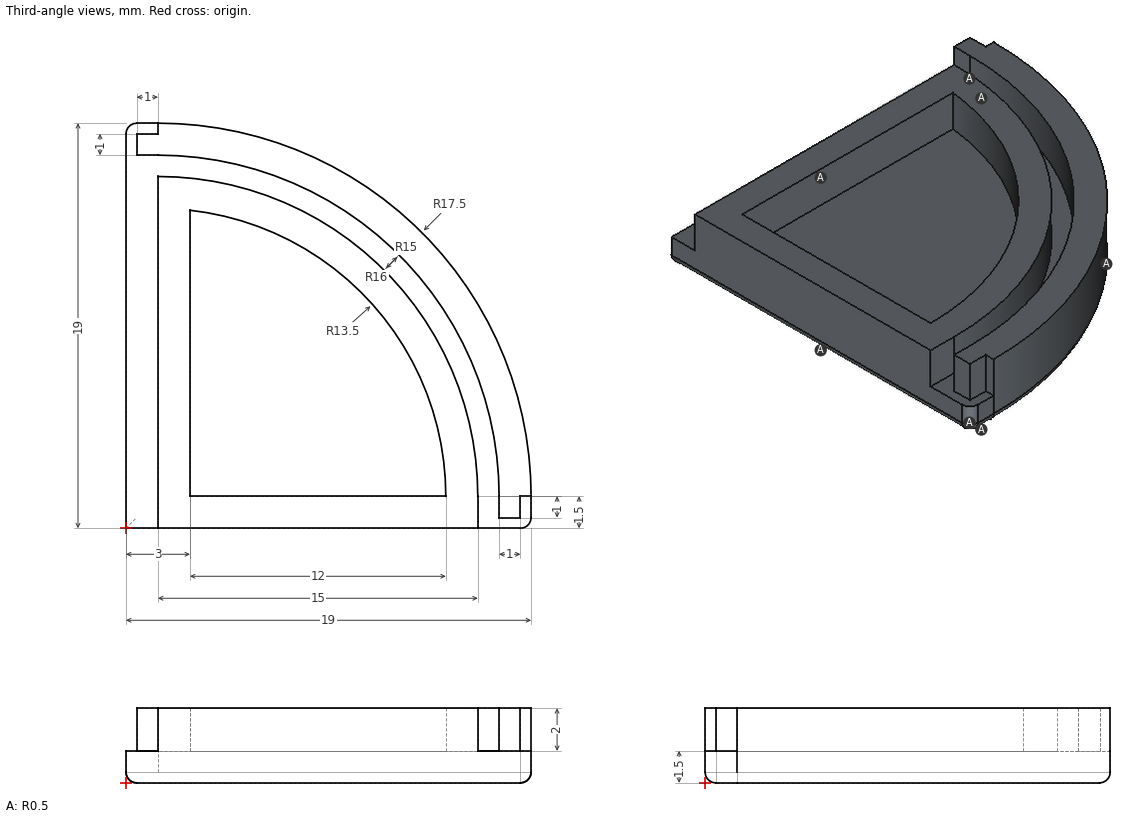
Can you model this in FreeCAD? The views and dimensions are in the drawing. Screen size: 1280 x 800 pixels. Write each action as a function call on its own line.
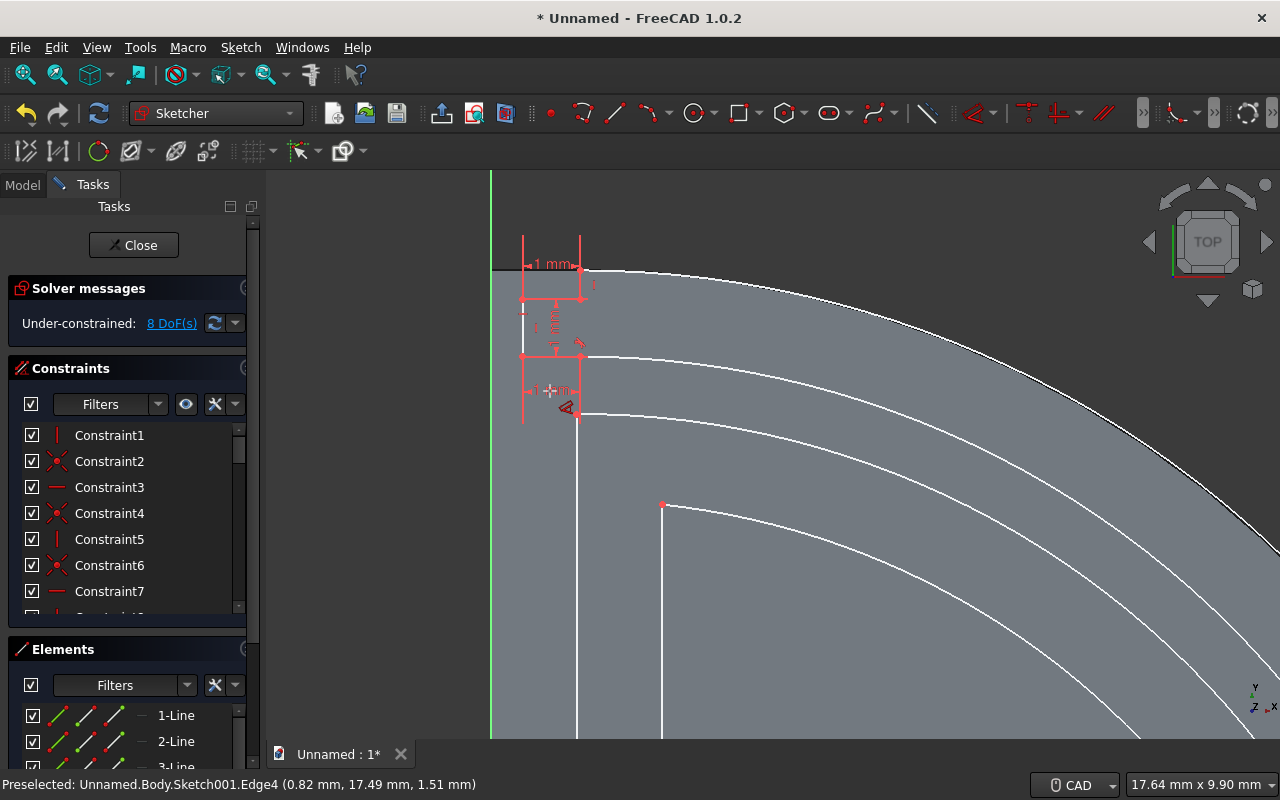
scroll(561, 299, down, 6)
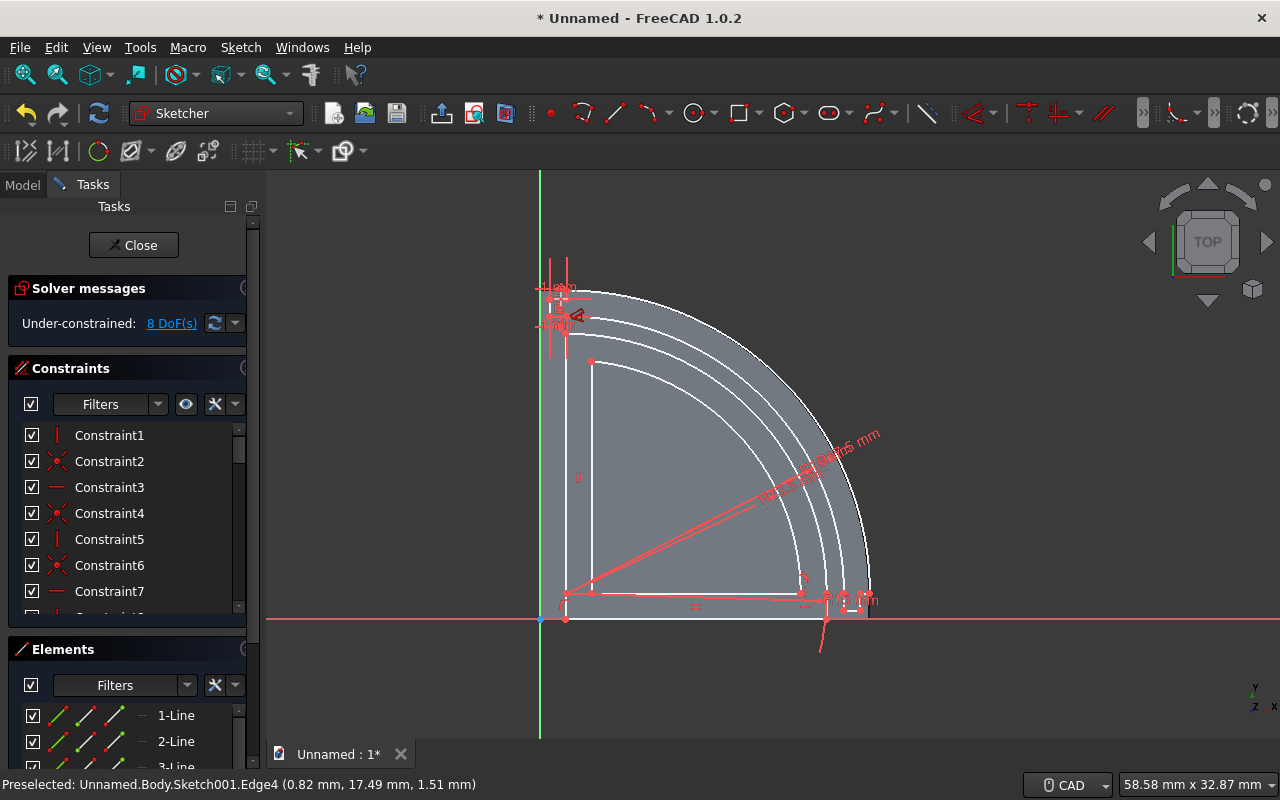
scroll(844, 599, up, 5)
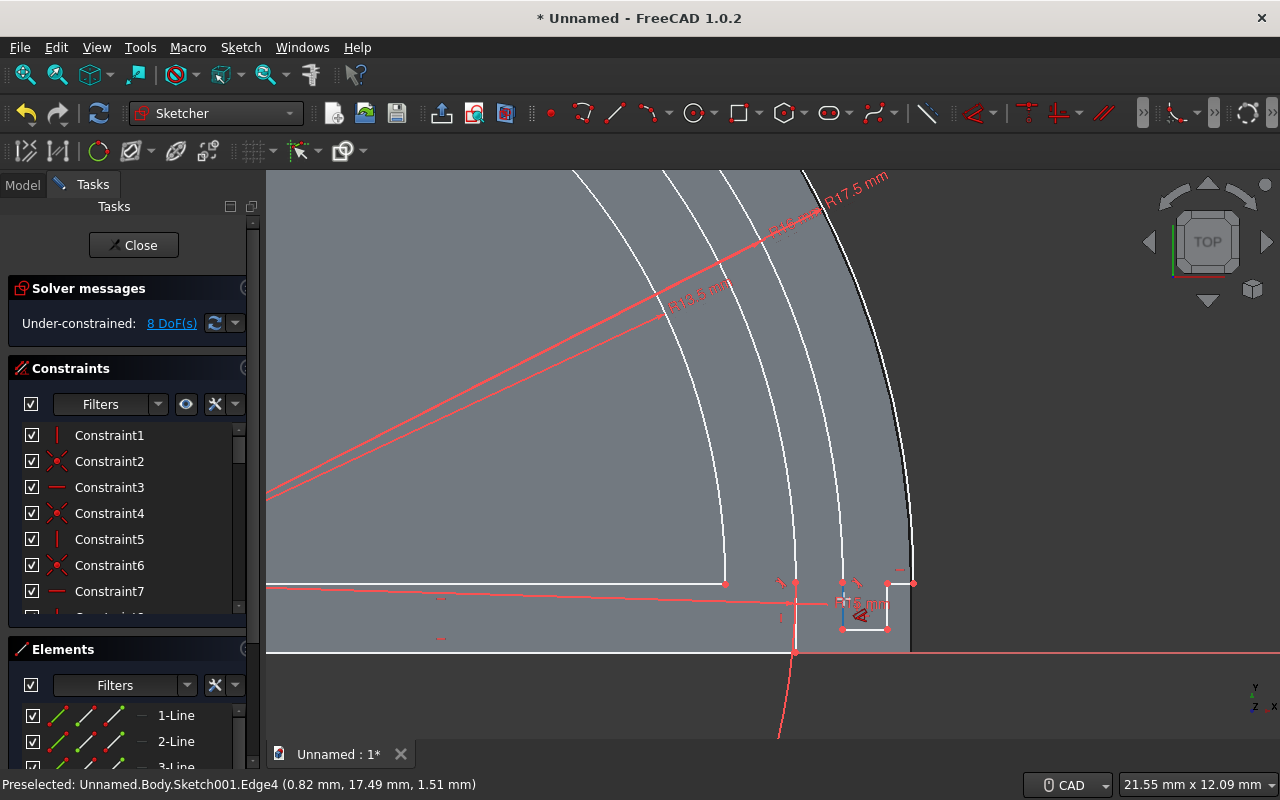
click(843, 597)
click(761, 606)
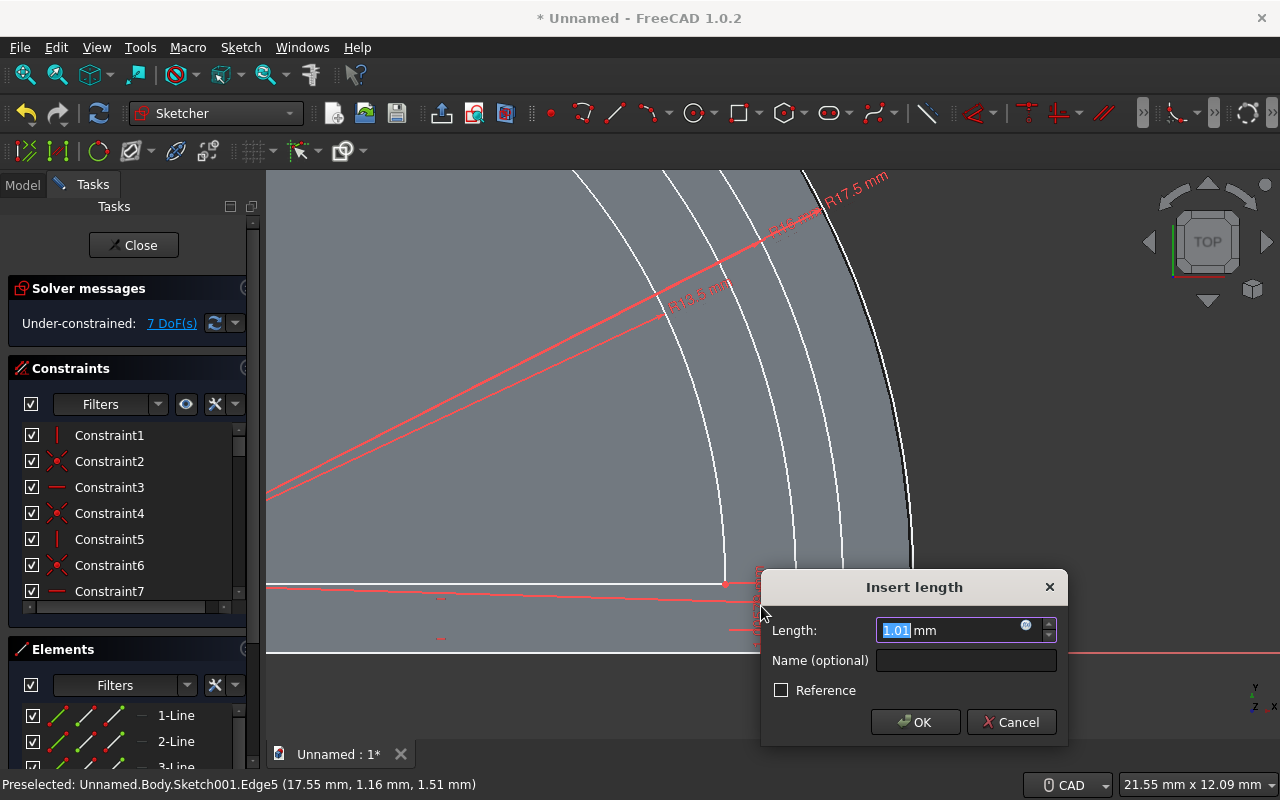
text(1)
key(Return)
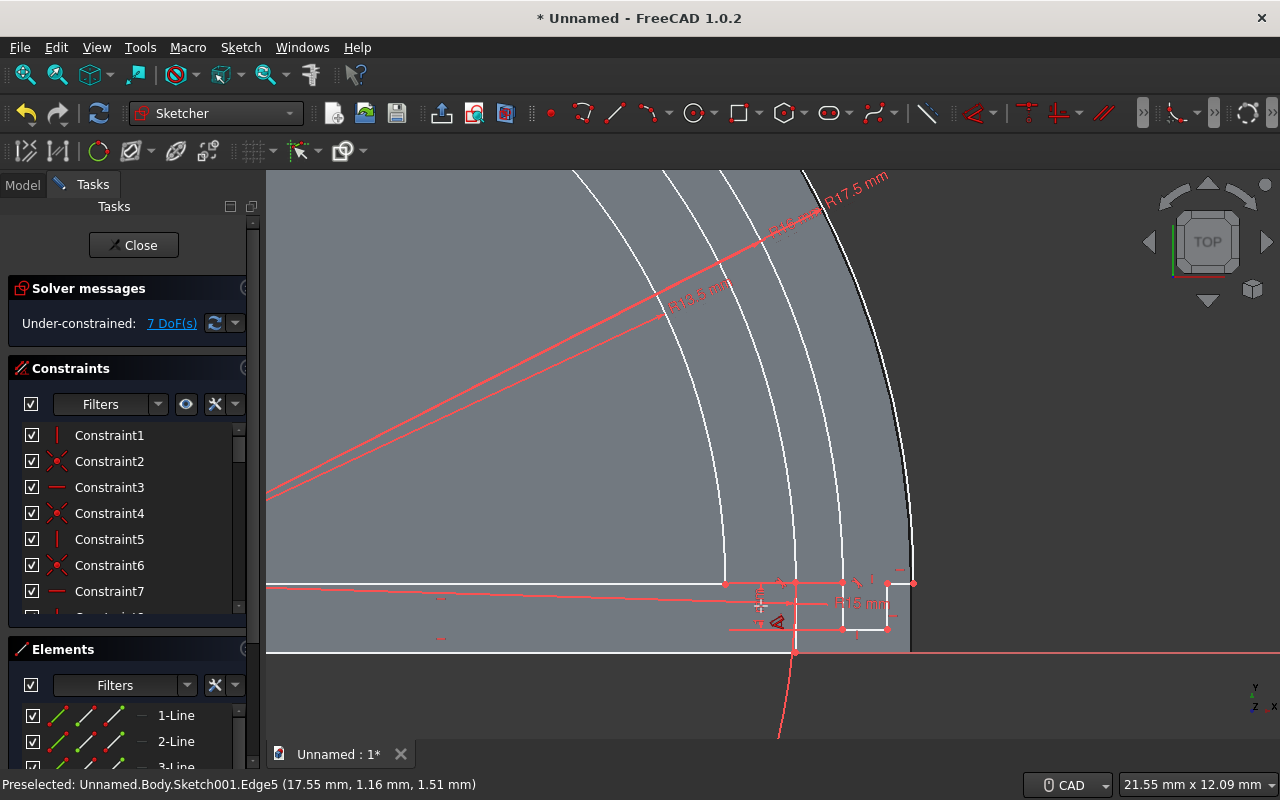
click(856, 630)
click(865, 688)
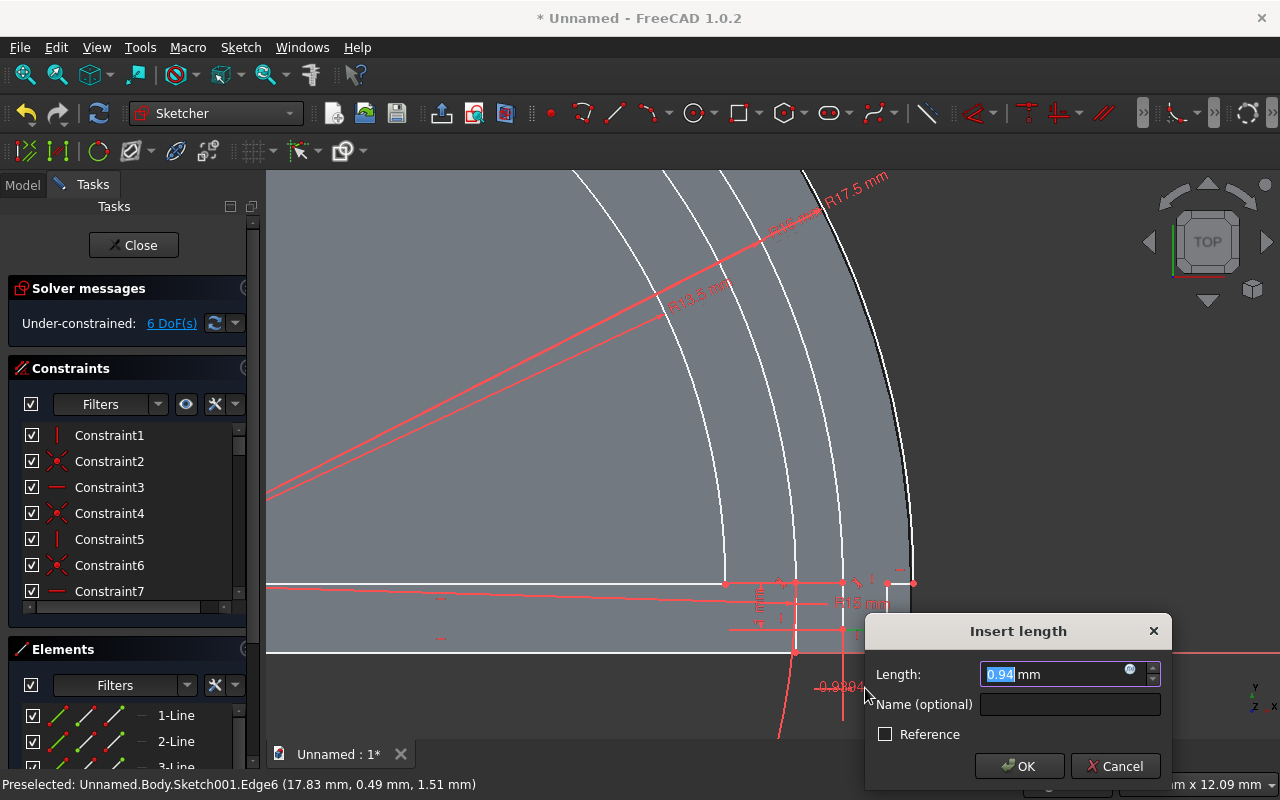
text(1)
key(Return)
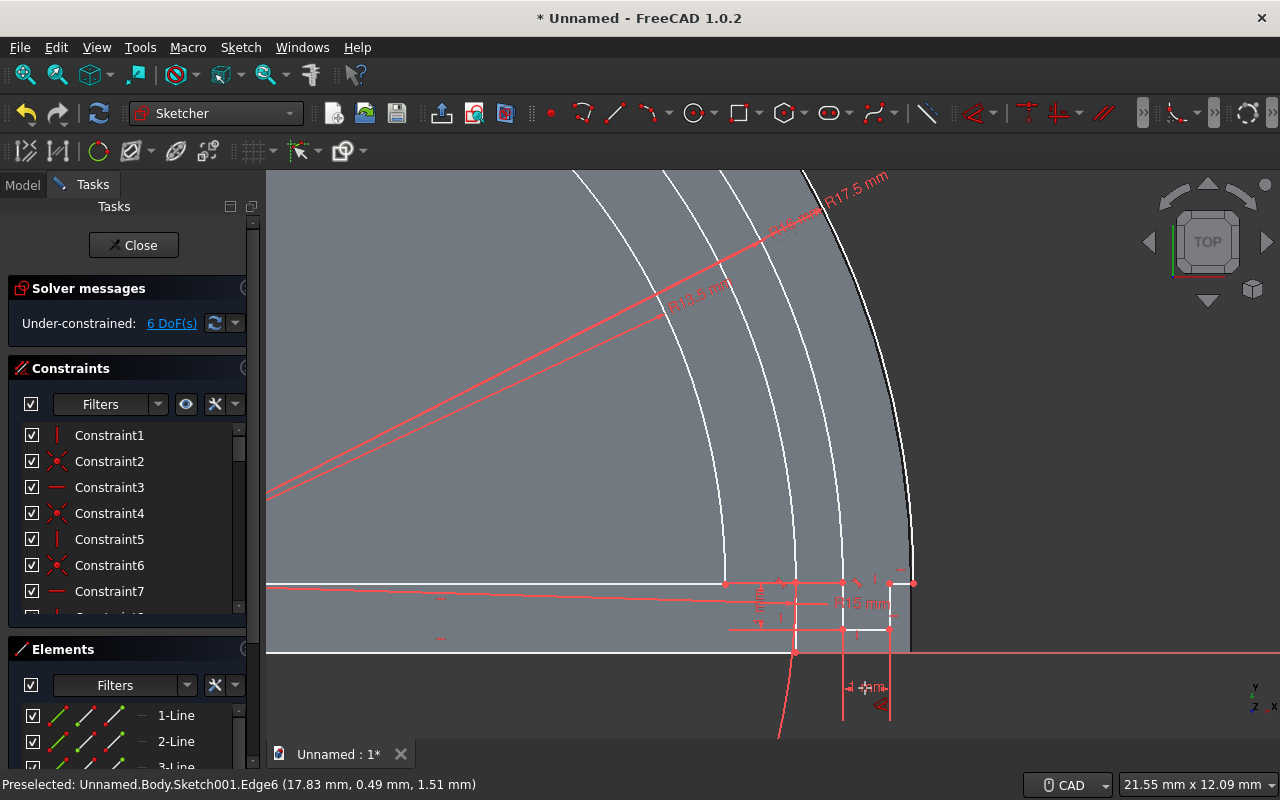
click(890, 616)
click(948, 607)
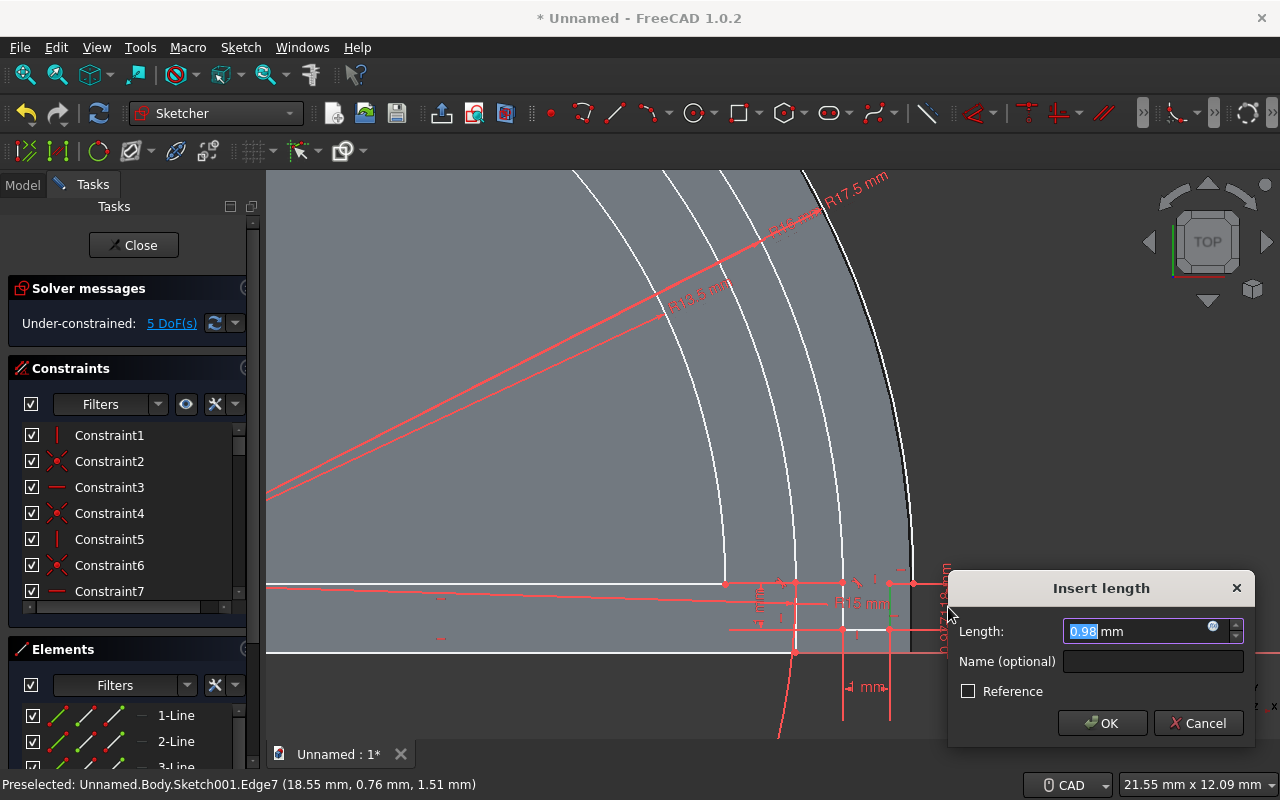
text(1)
key(Return)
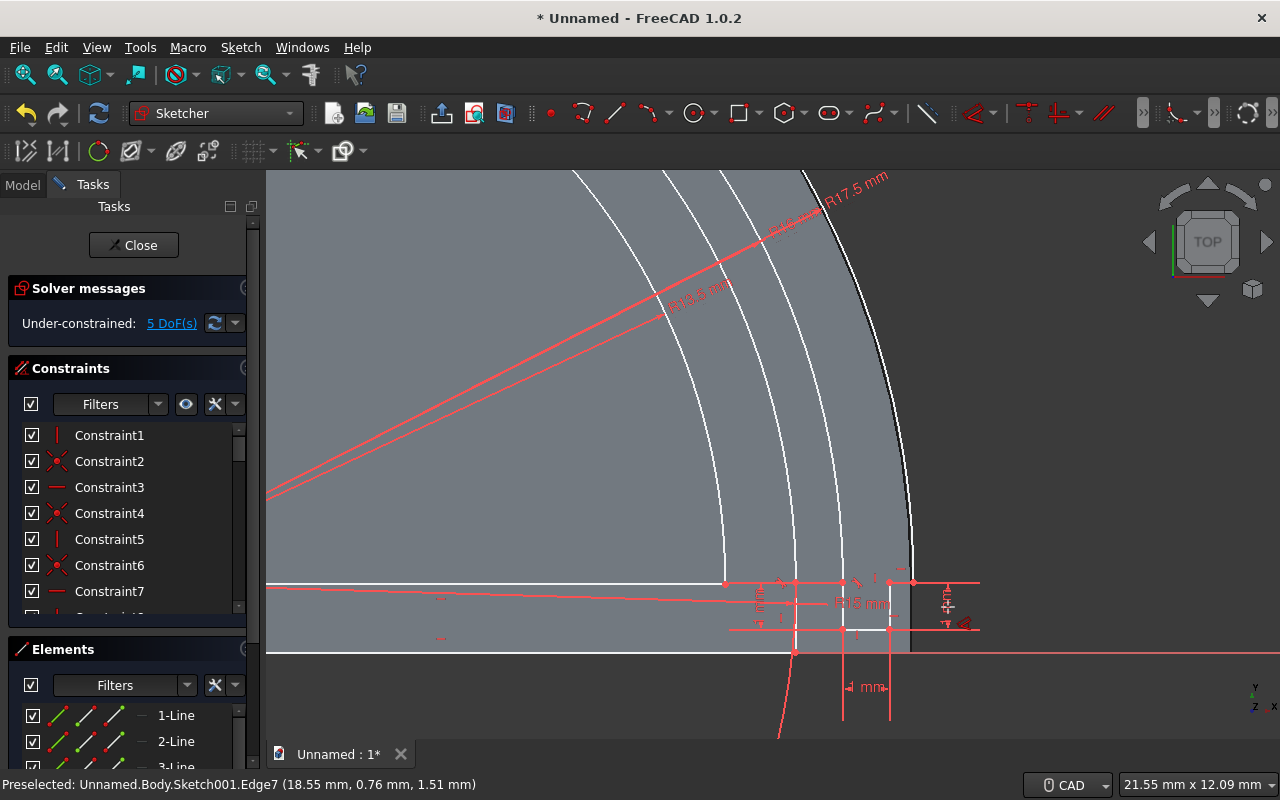
click(300, 653)
click(545, 687)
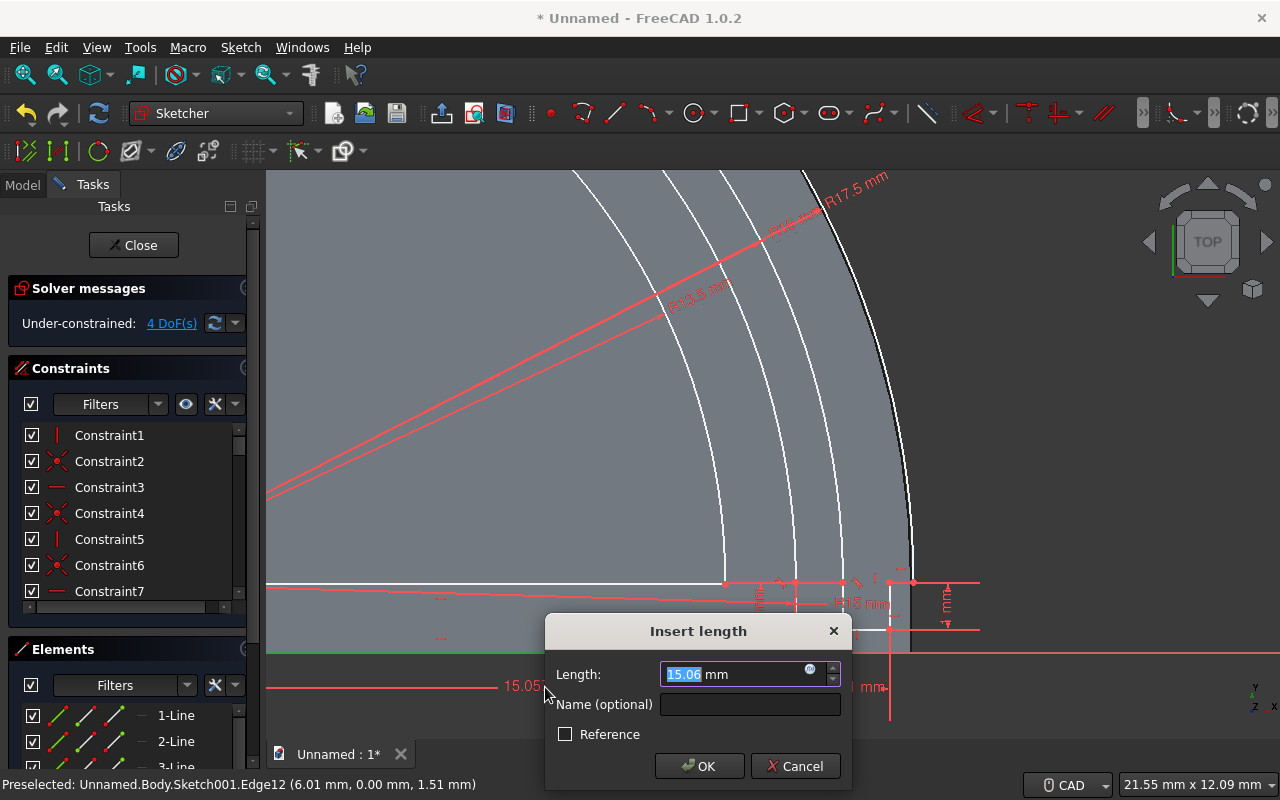
text(15)
key(Return)